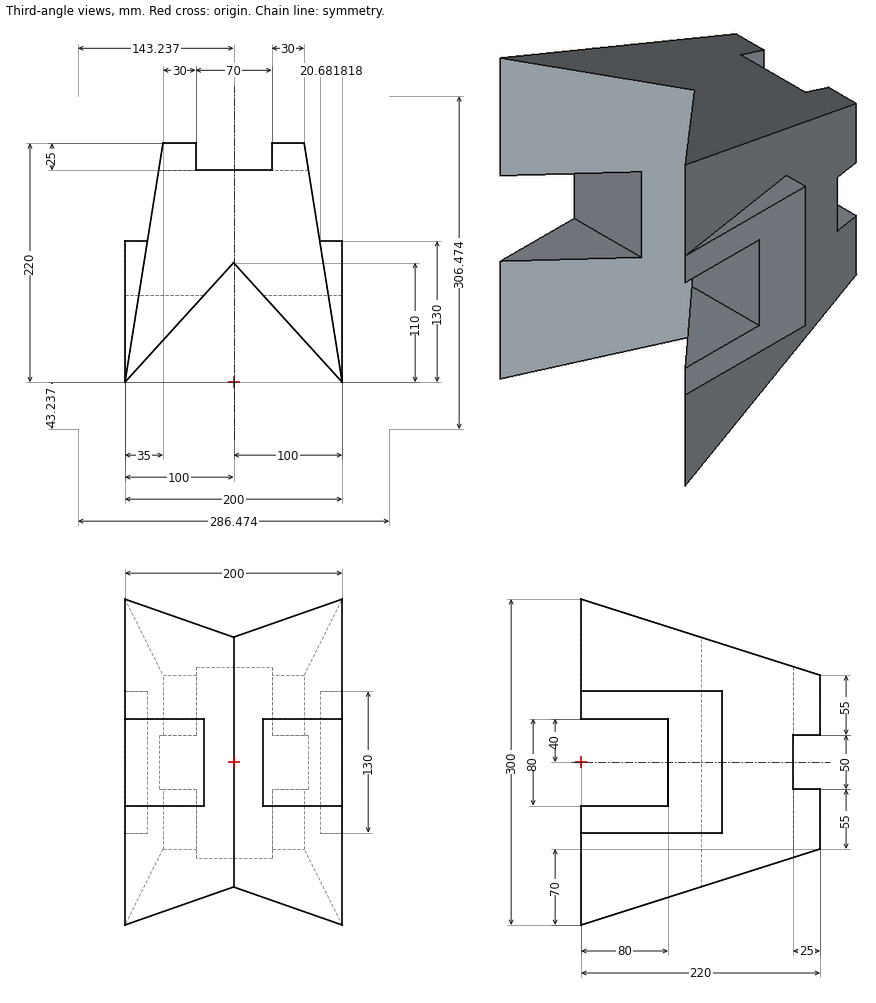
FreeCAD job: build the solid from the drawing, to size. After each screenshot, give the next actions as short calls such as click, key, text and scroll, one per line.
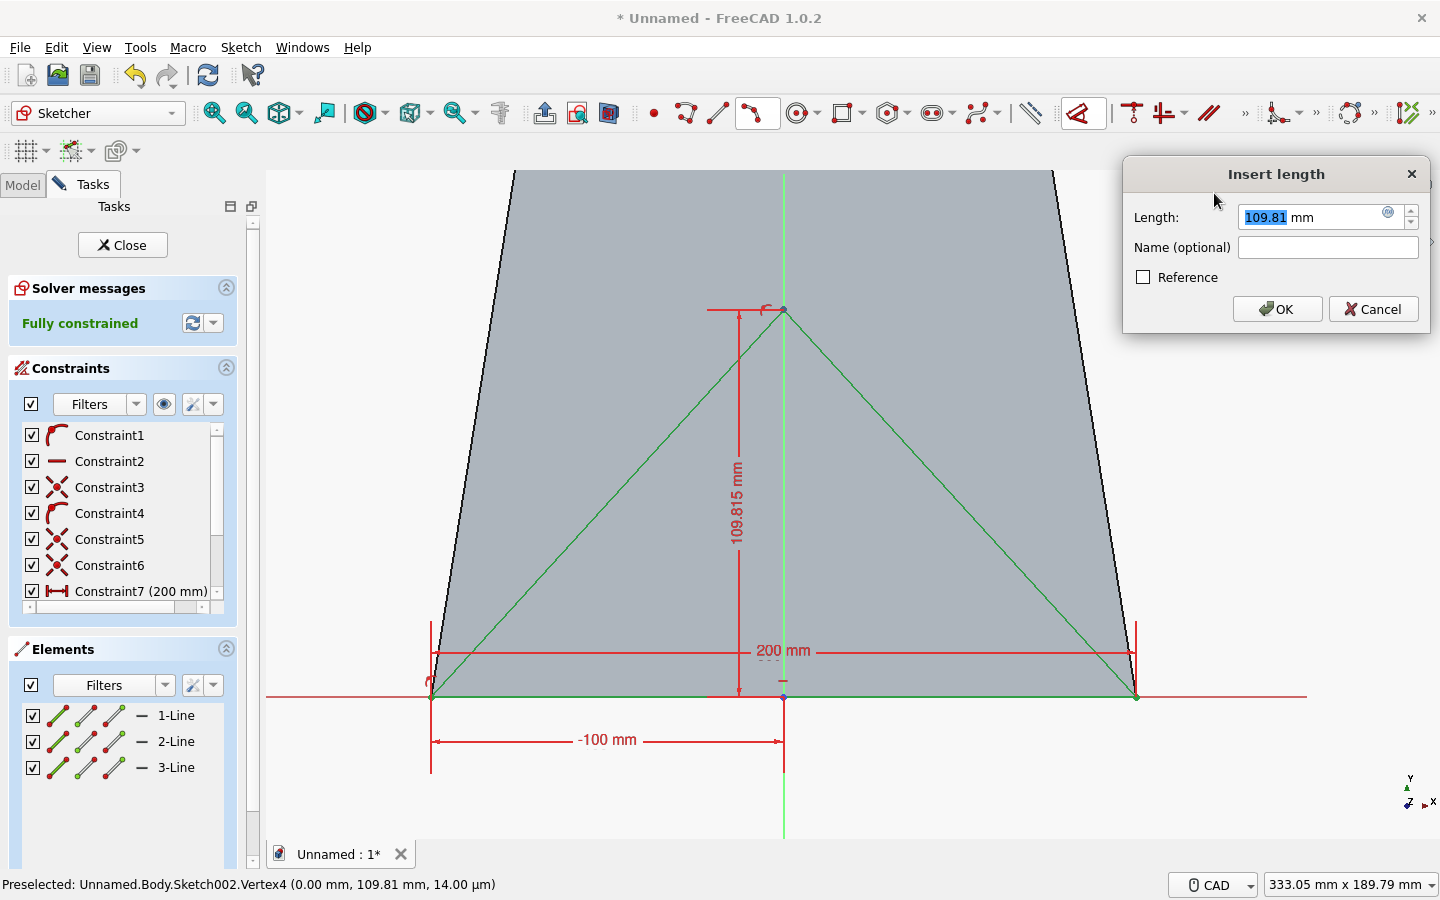
text(110)
key(Return)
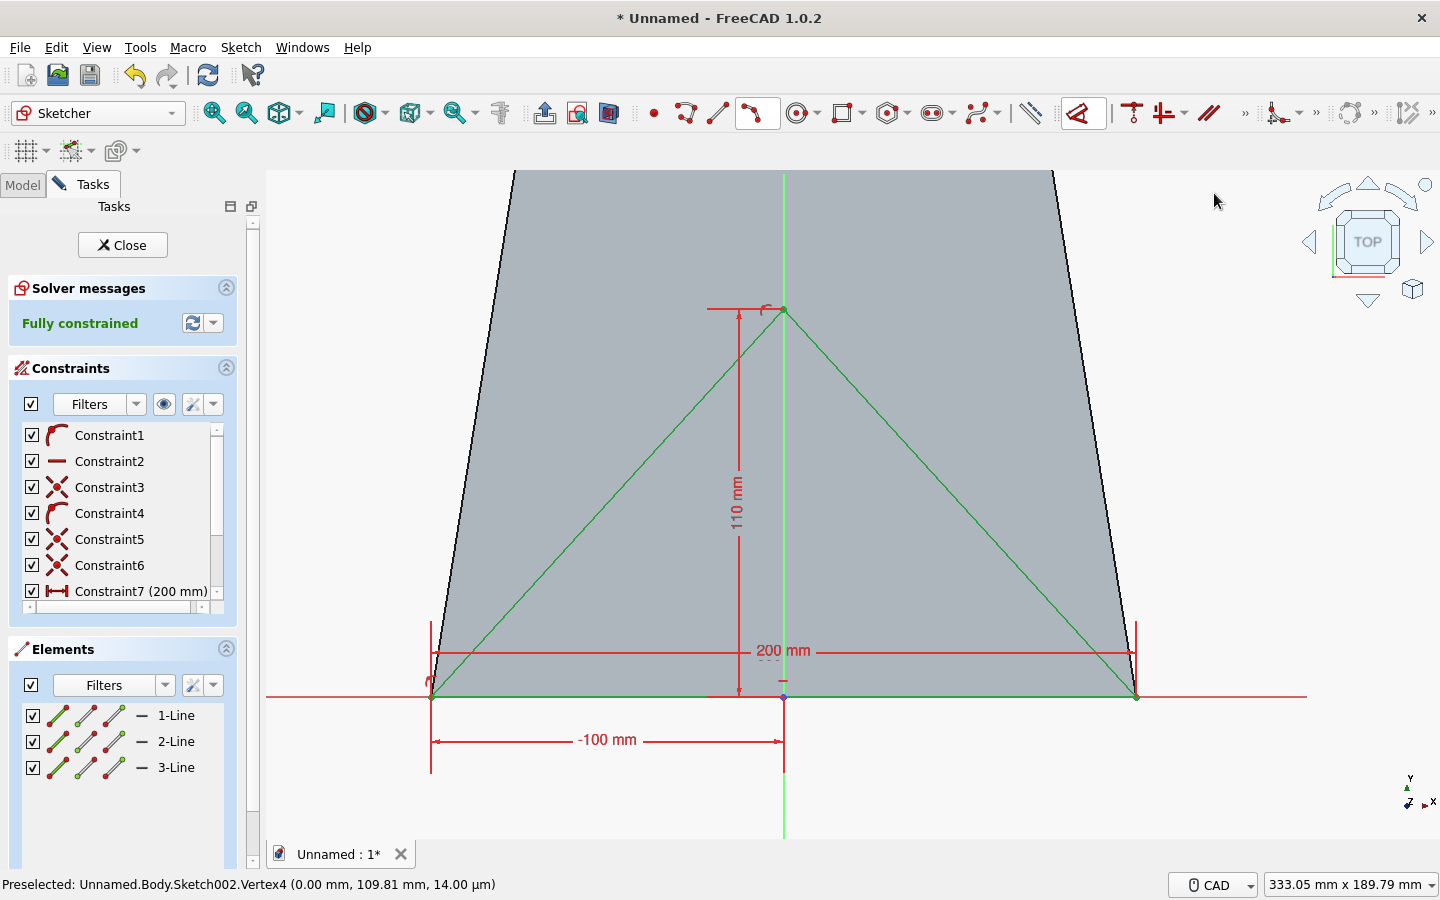
click(123, 245)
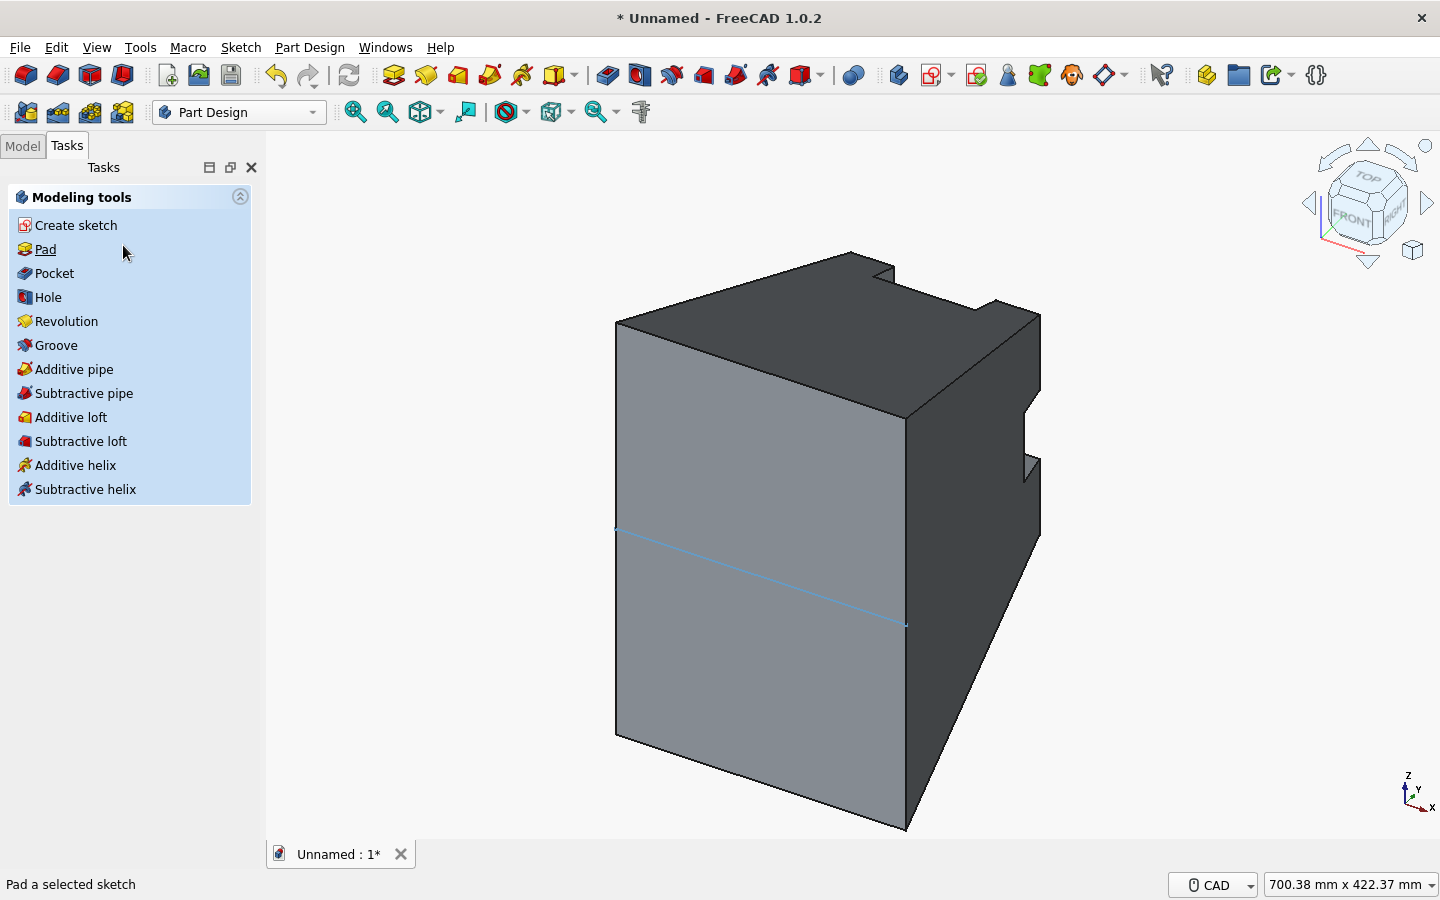
click(608, 76)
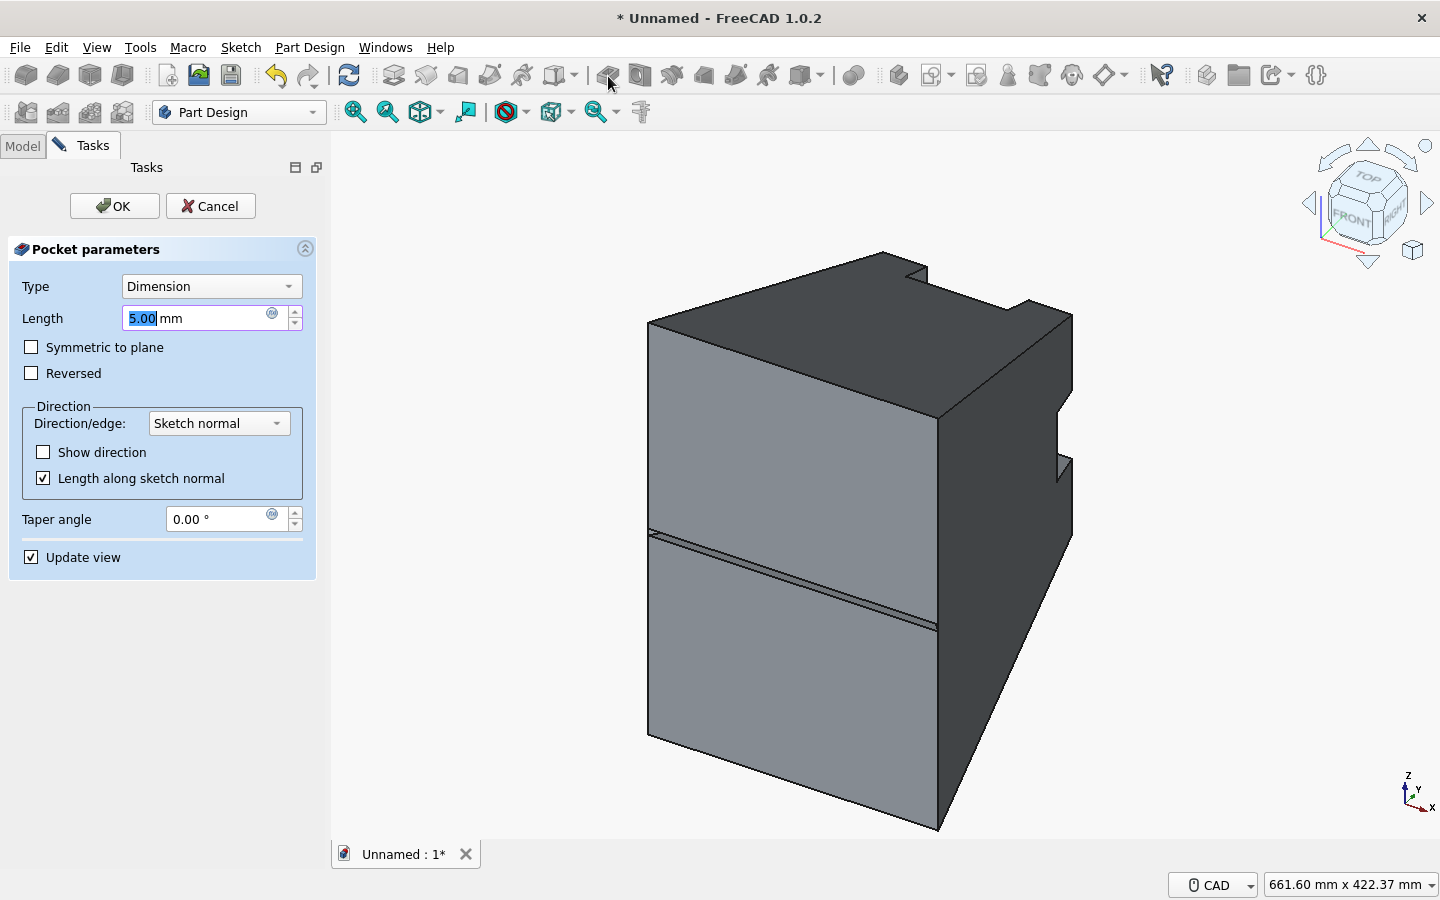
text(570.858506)
key(Tab)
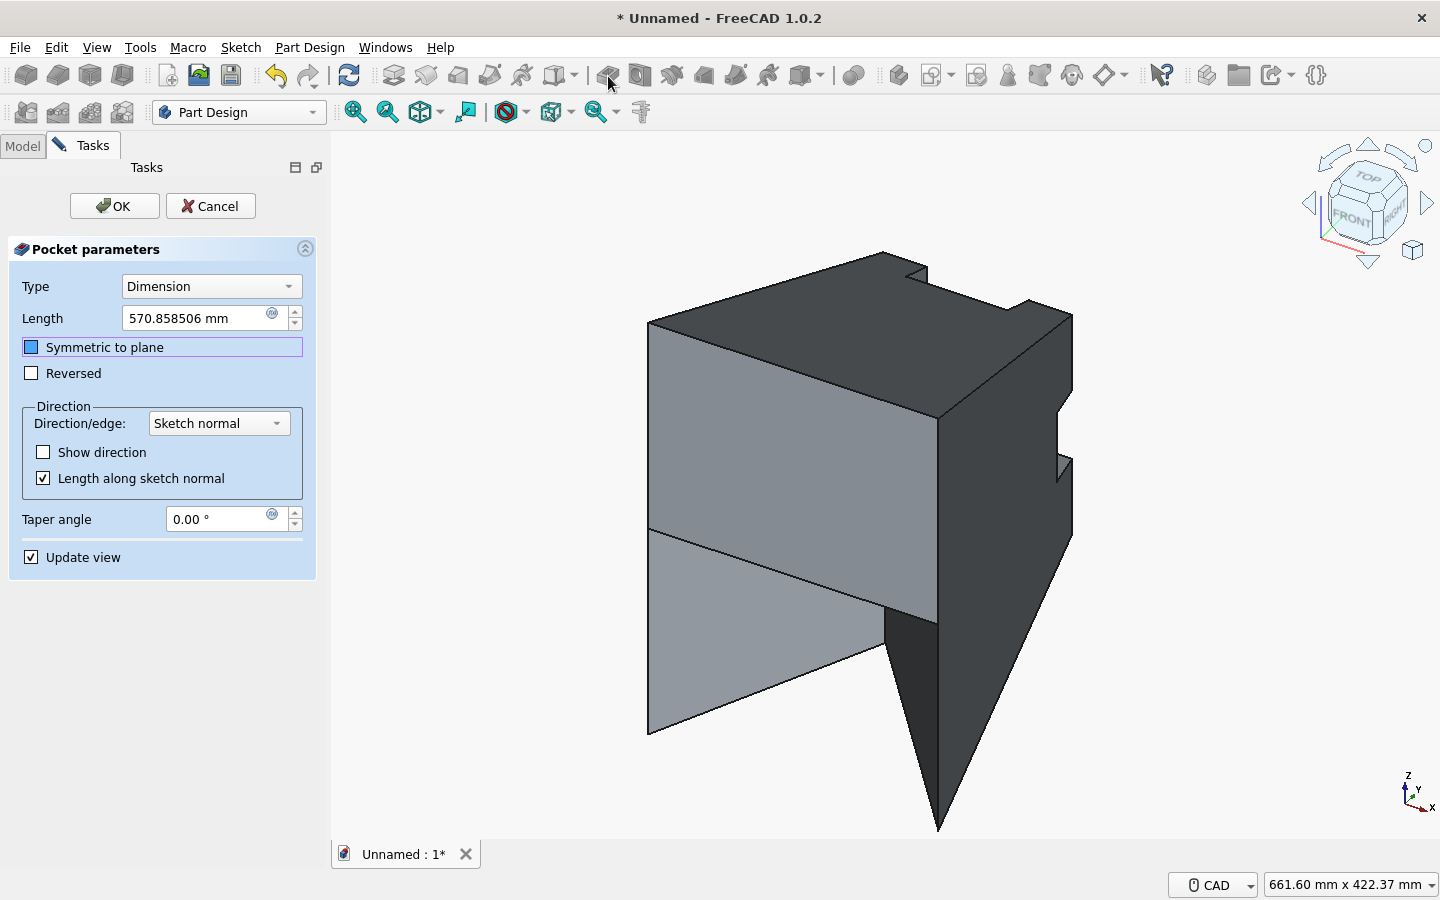
click(30, 347)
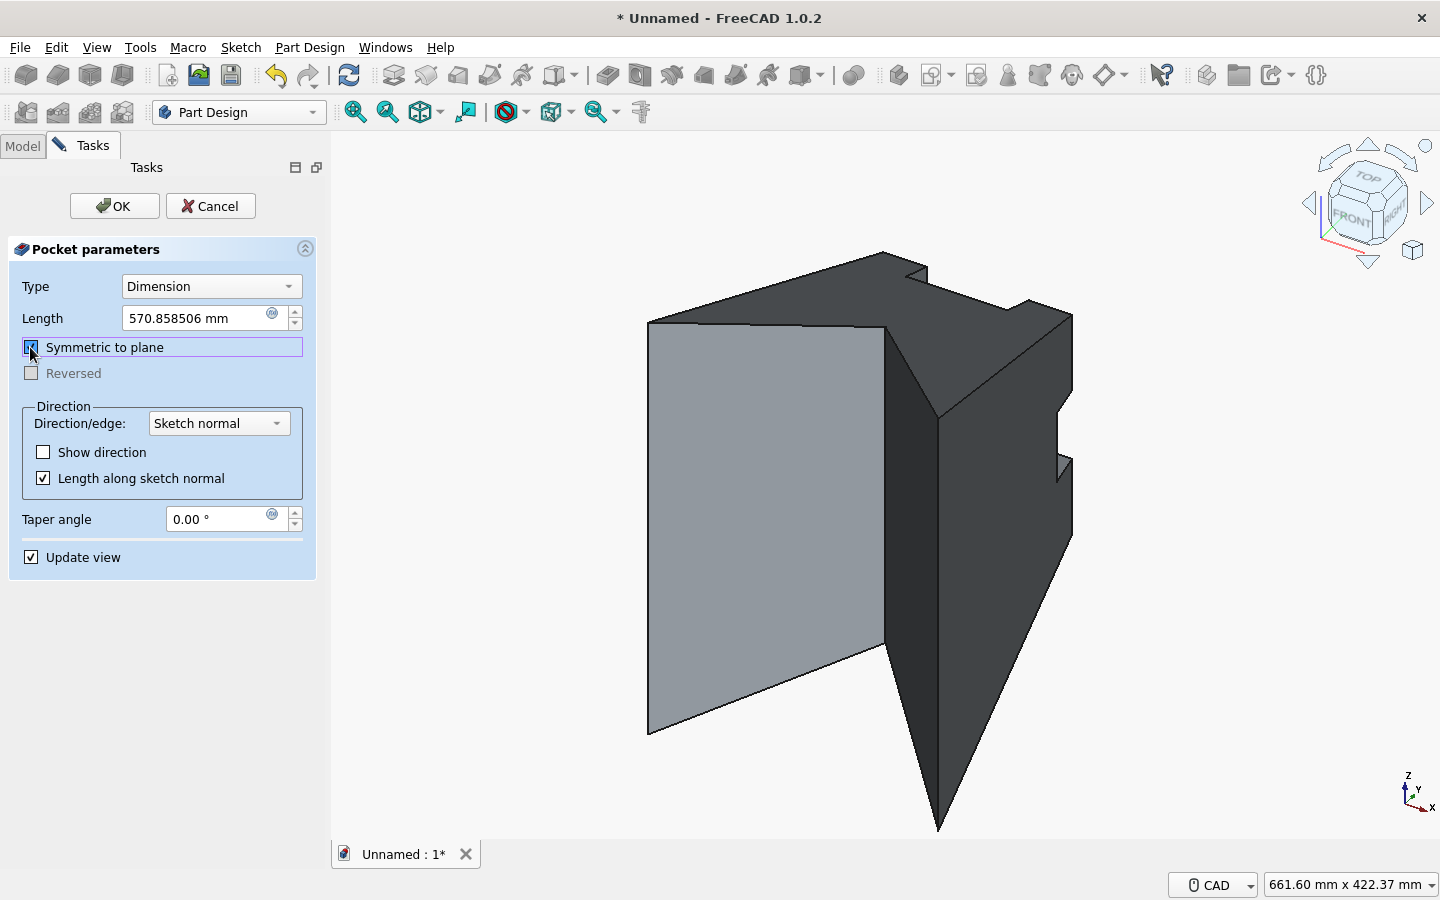
click(115, 206)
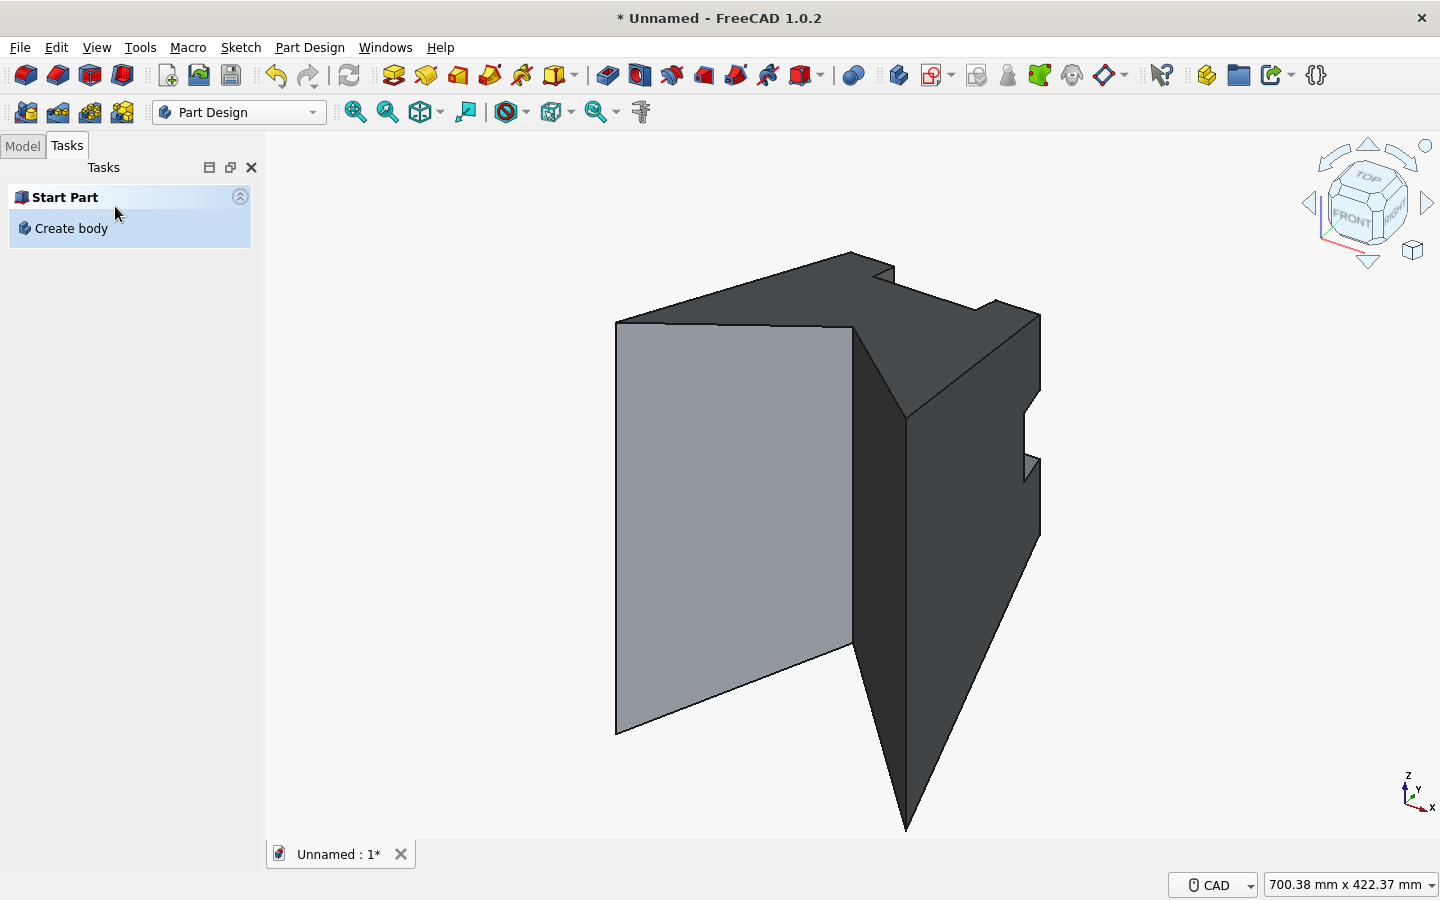
click(932, 76)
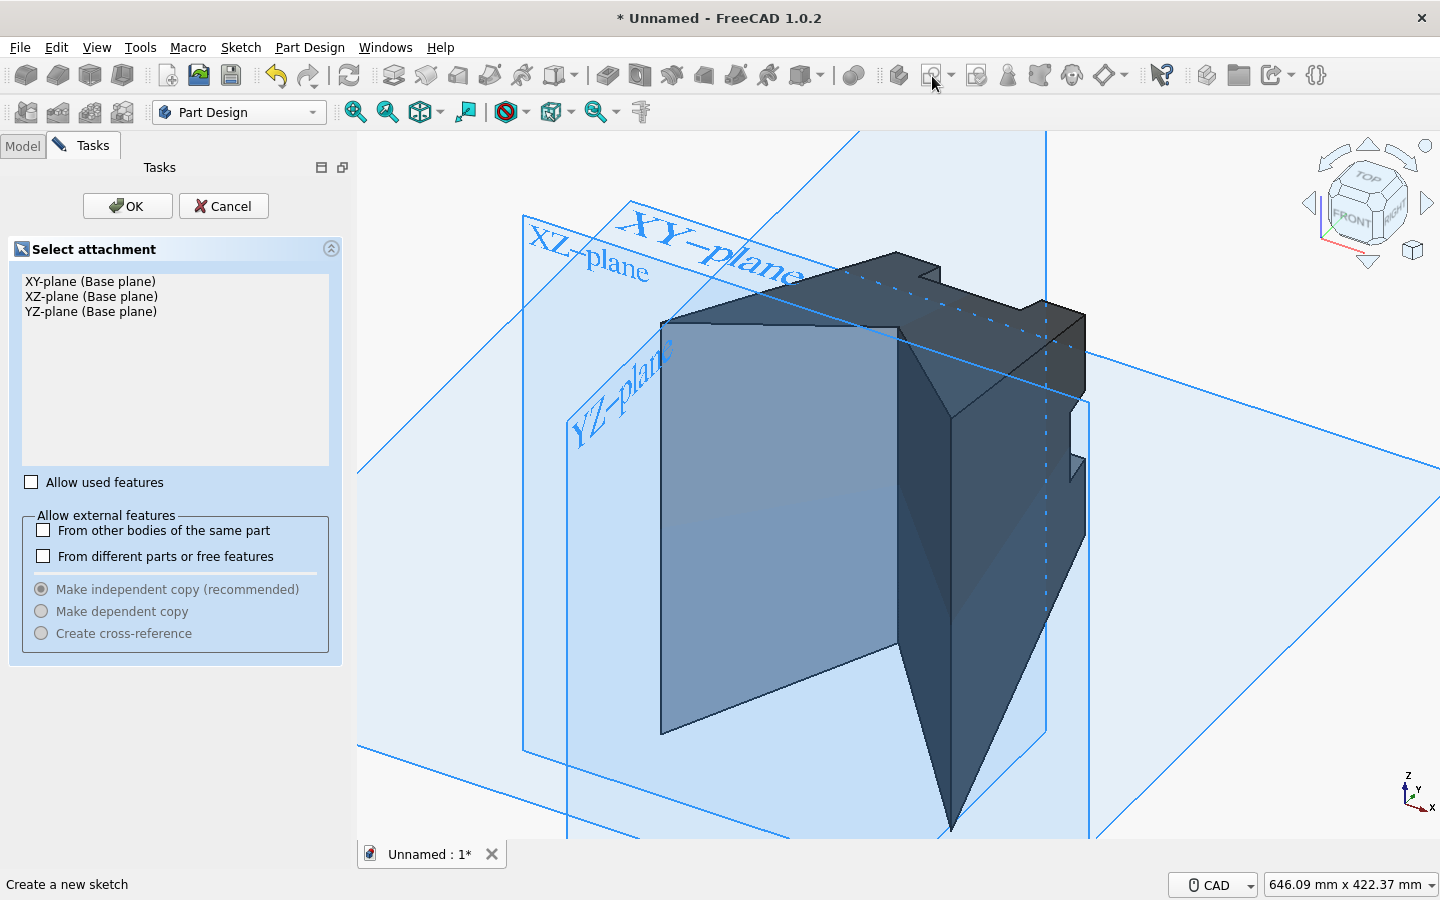
click(82, 282)